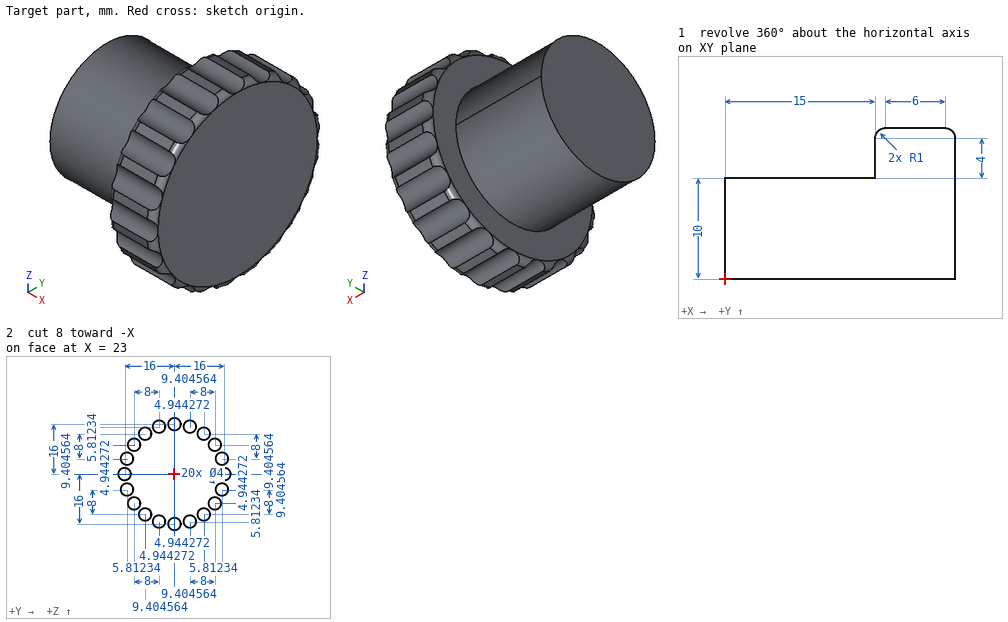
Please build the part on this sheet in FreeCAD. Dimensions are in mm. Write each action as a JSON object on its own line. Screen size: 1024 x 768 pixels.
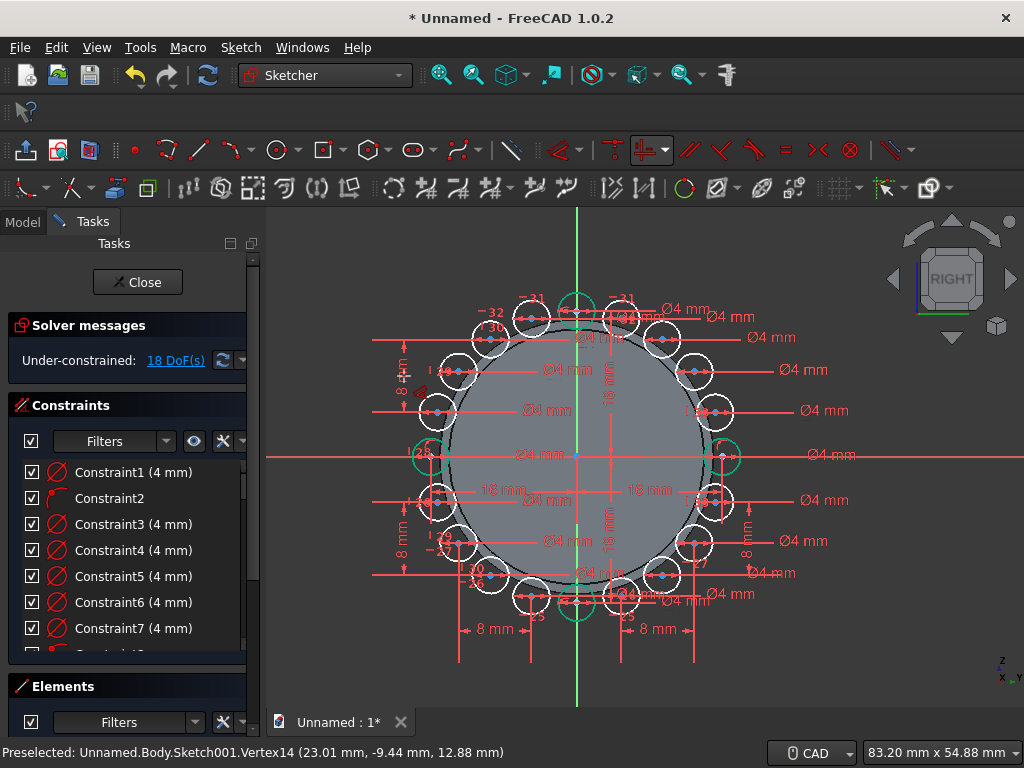
{"action": "left_click", "coordinate": [459, 372]}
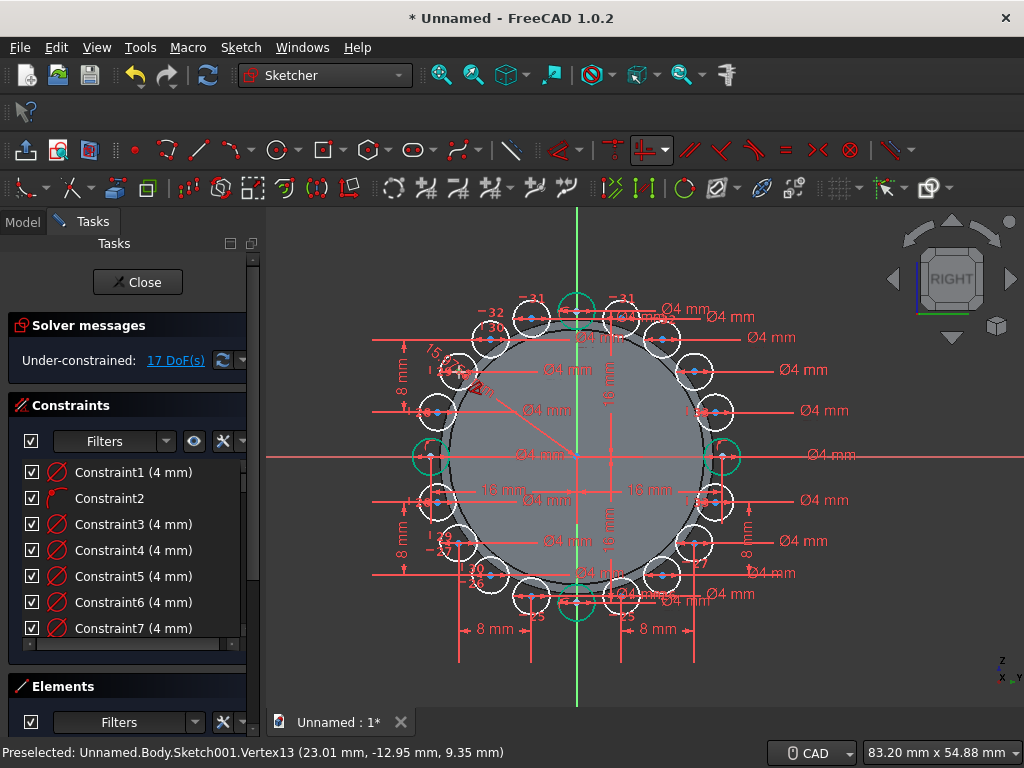
{"action": "left_click", "coordinate": [532, 319]}
{"action": "left_click", "coordinate": [495, 285]}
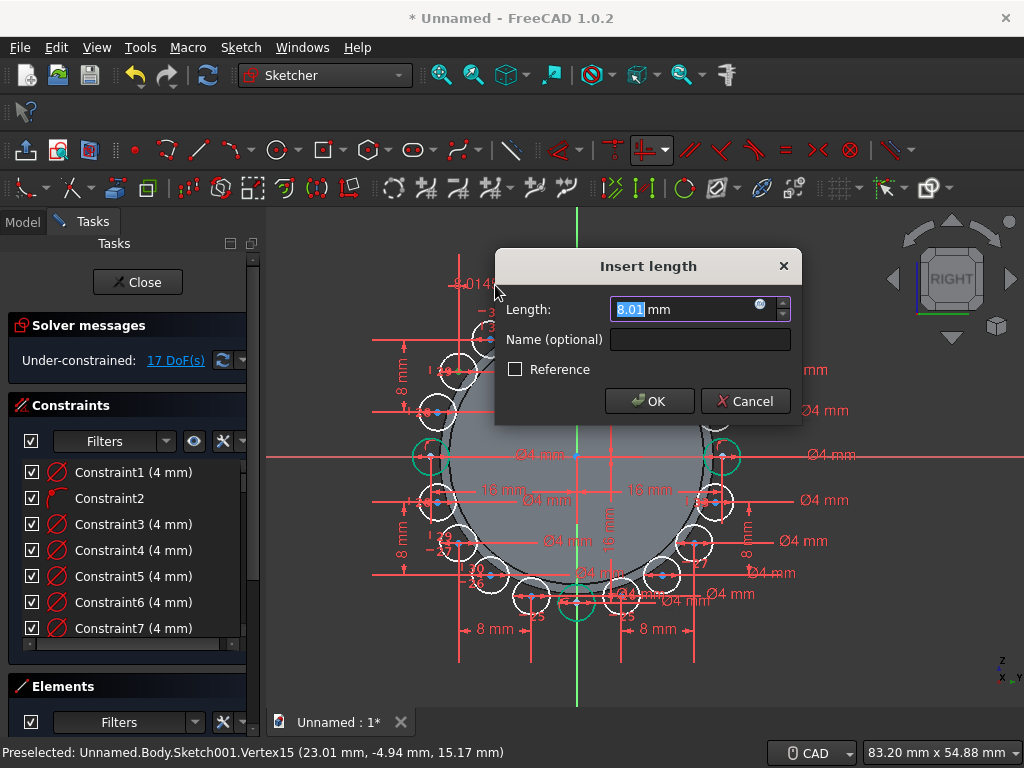
{"action": "type", "text": "8"}
{"action": "key", "text": "Return"}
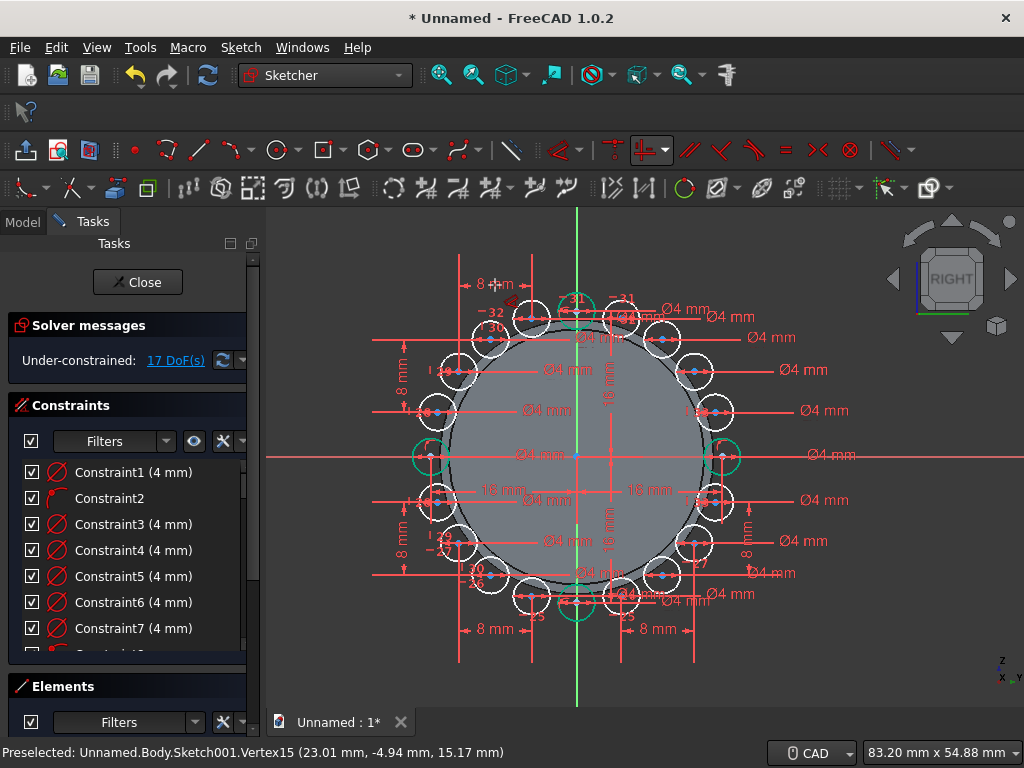
{"action": "left_click", "coordinate": [621, 319]}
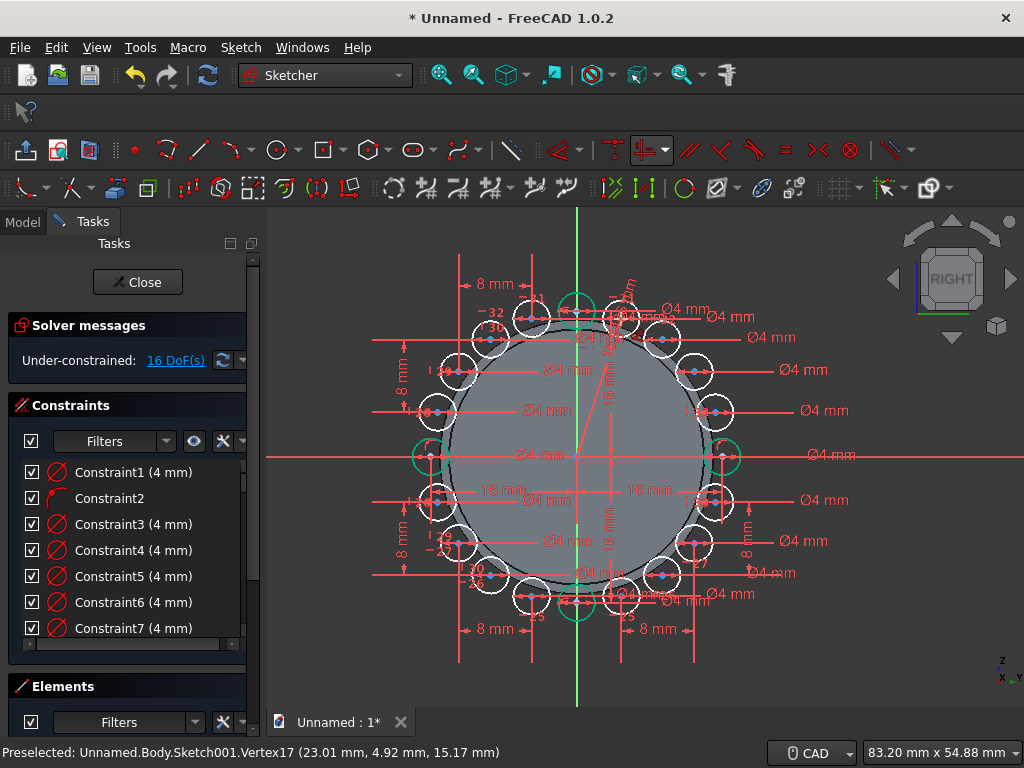
{"action": "left_click", "coordinate": [694, 372]}
{"action": "left_click", "coordinate": [658, 285]}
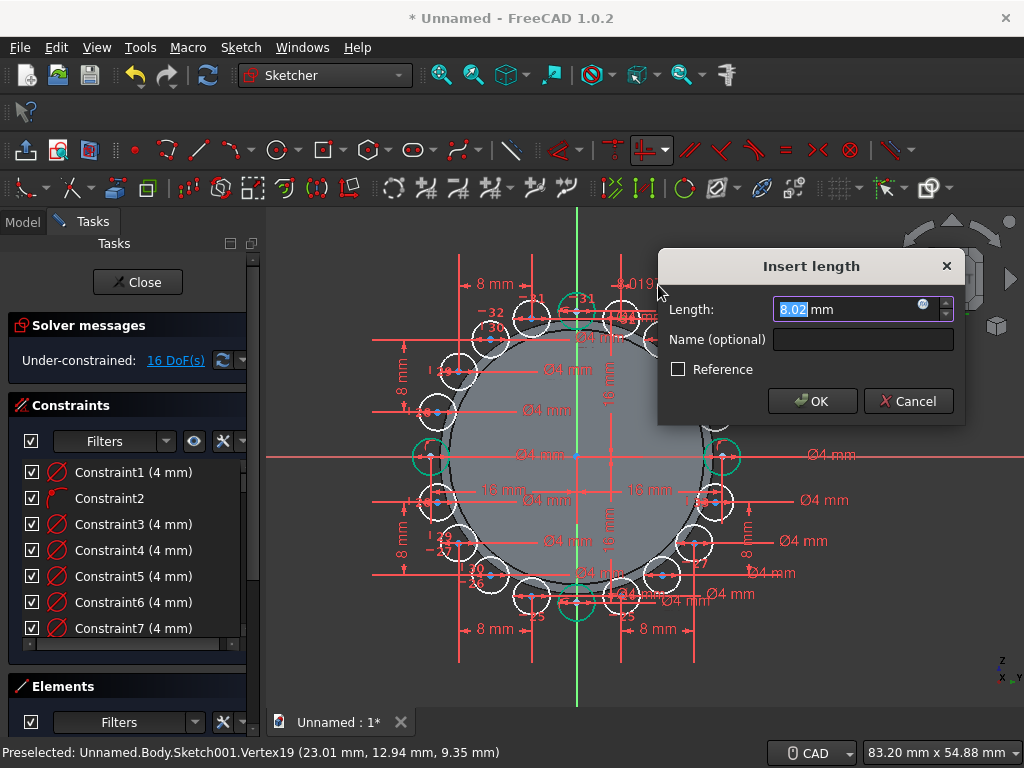
{"action": "type", "text": "8"}
{"action": "key", "text": "Return"}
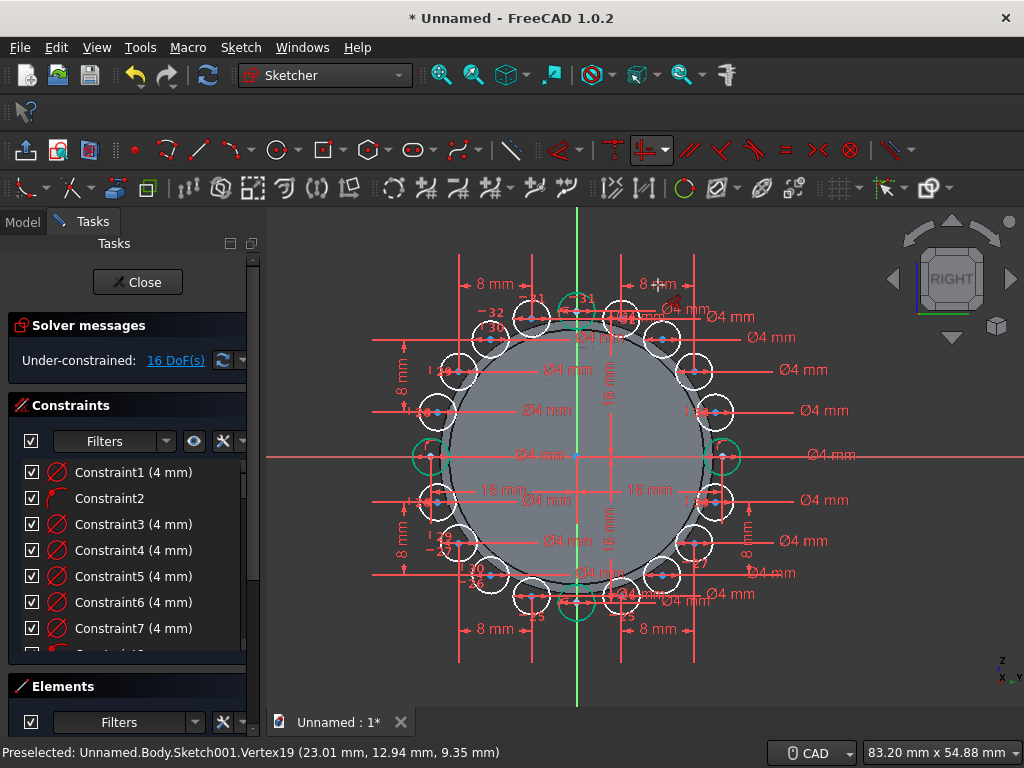
{"action": "left_click", "coordinate": [662, 340]}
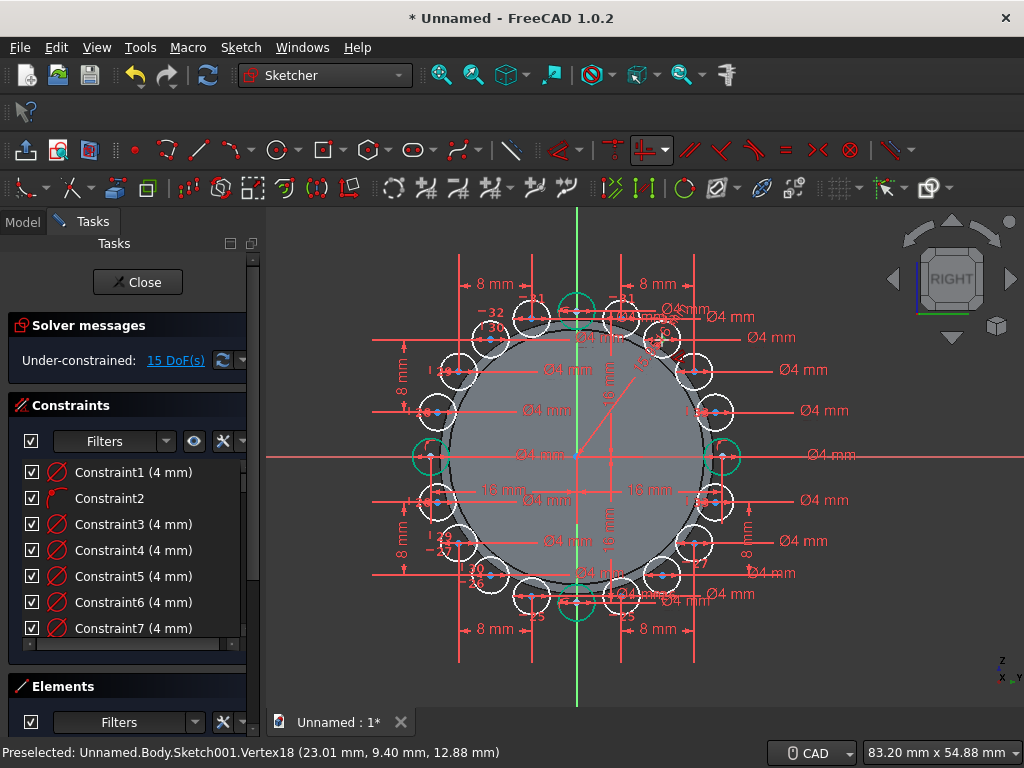
{"action": "left_click", "coordinate": [715, 413]}
{"action": "left_click", "coordinate": [749, 376]}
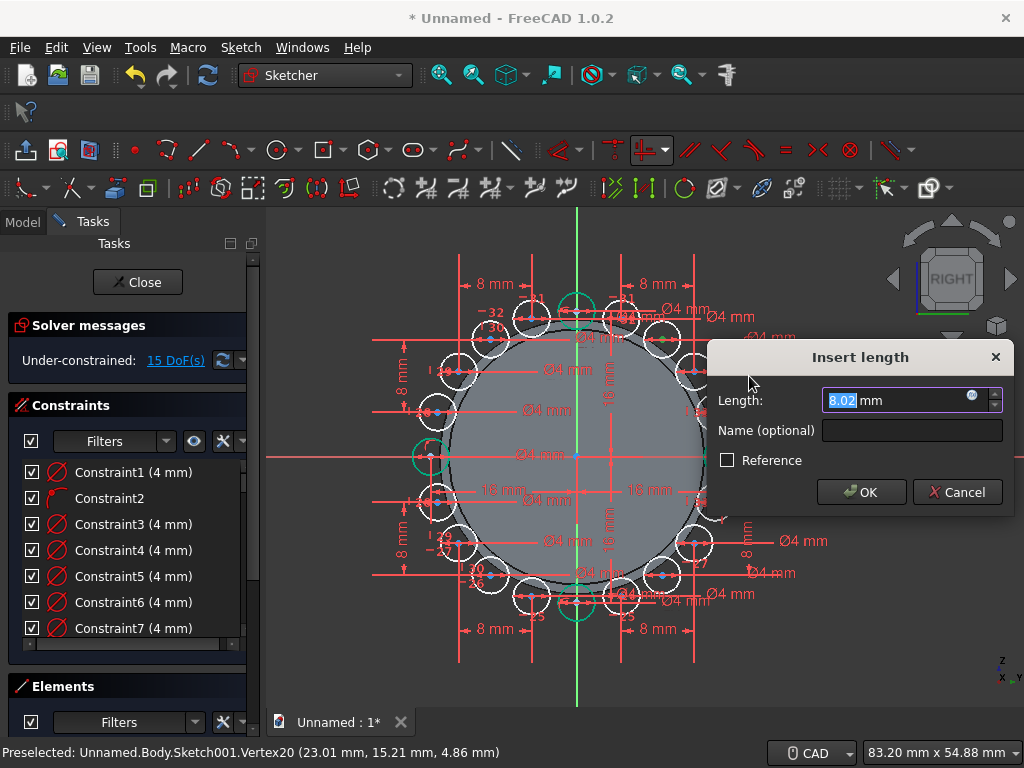
{"action": "type", "text": "8"}
{"action": "key", "text": "Return"}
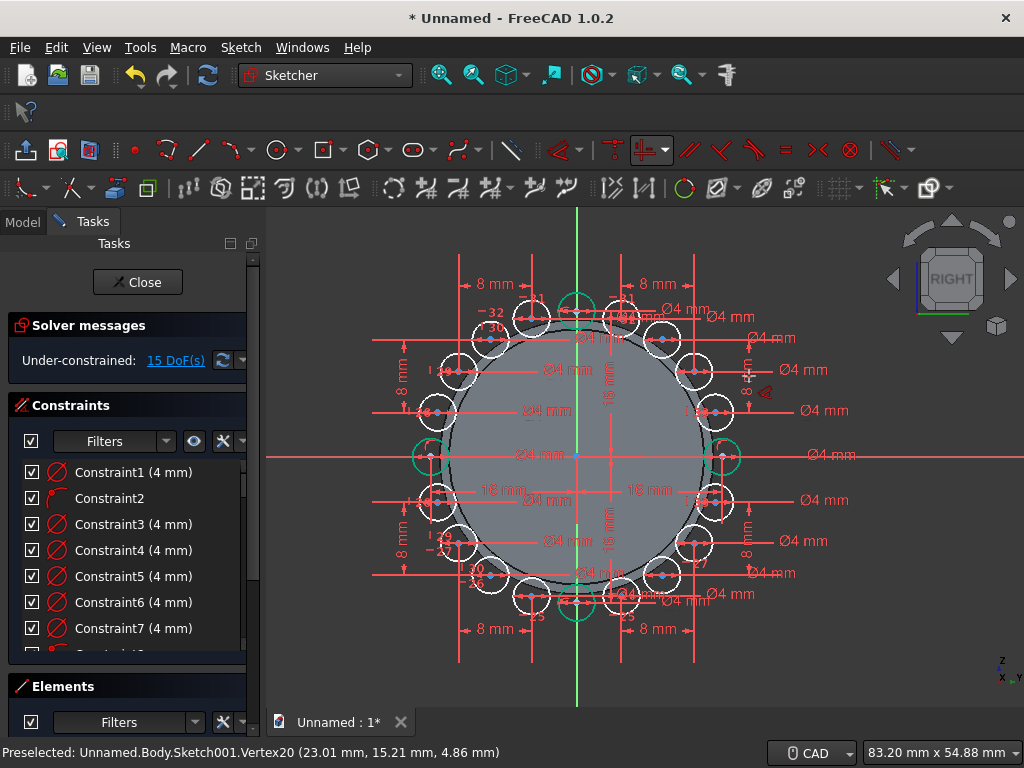
{"action": "left_click", "coordinate": [715, 502]}
{"action": "left_click", "coordinate": [749, 480]}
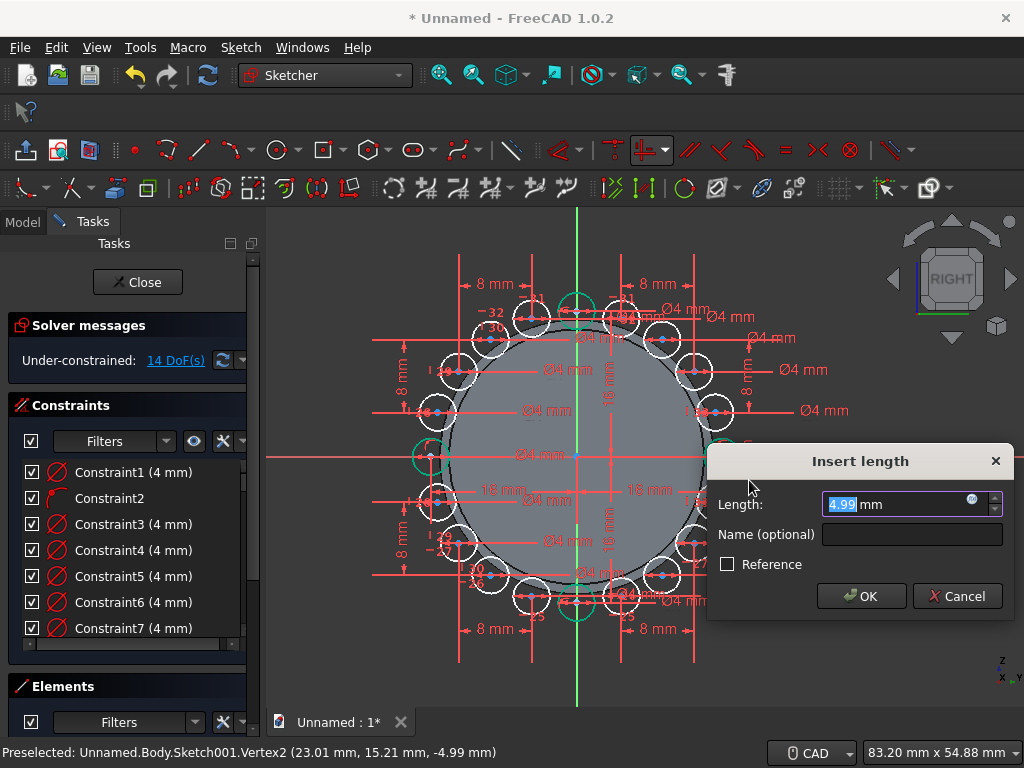
{"action": "type", "text": "4.944272"}
{"action": "key", "text": "Return"}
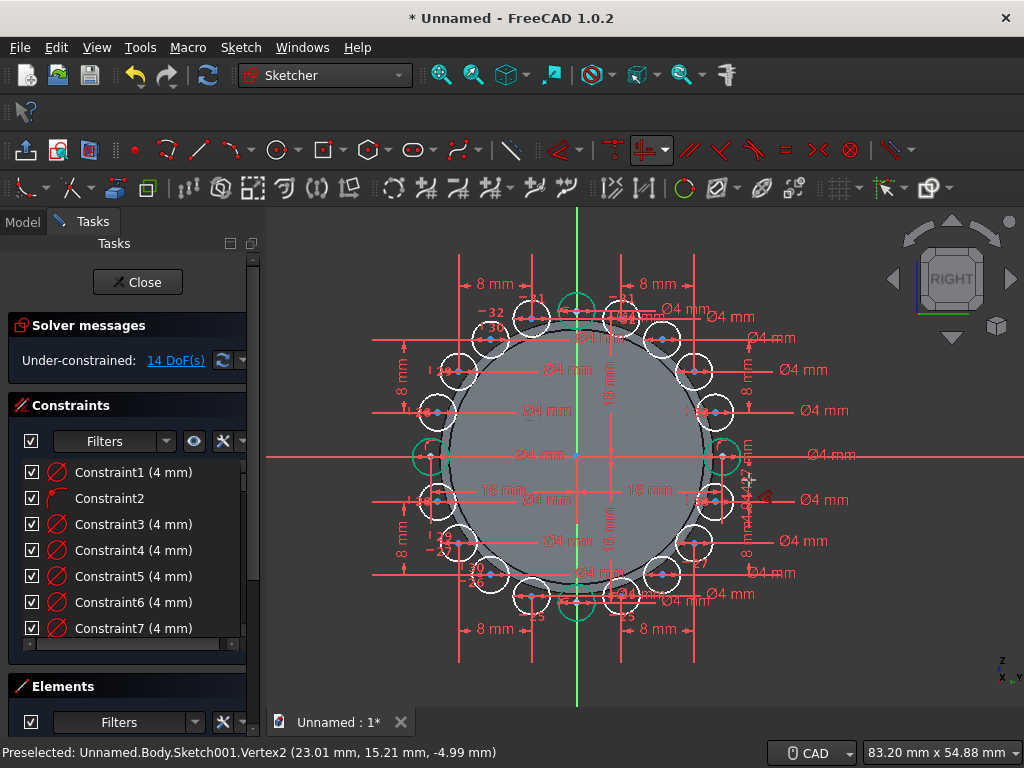
{"action": "left_click", "coordinate": [694, 543]}
{"action": "left_click", "coordinate": [752, 500]}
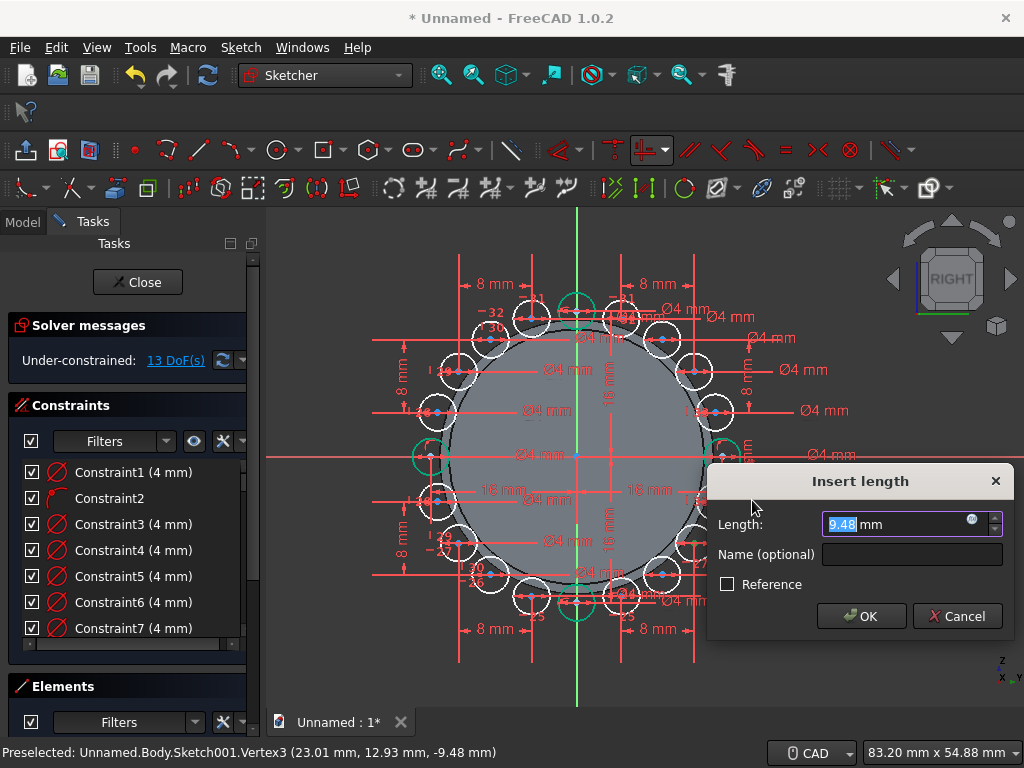
{"action": "type", "text": "9.404564"}
{"action": "key", "text": "Return"}